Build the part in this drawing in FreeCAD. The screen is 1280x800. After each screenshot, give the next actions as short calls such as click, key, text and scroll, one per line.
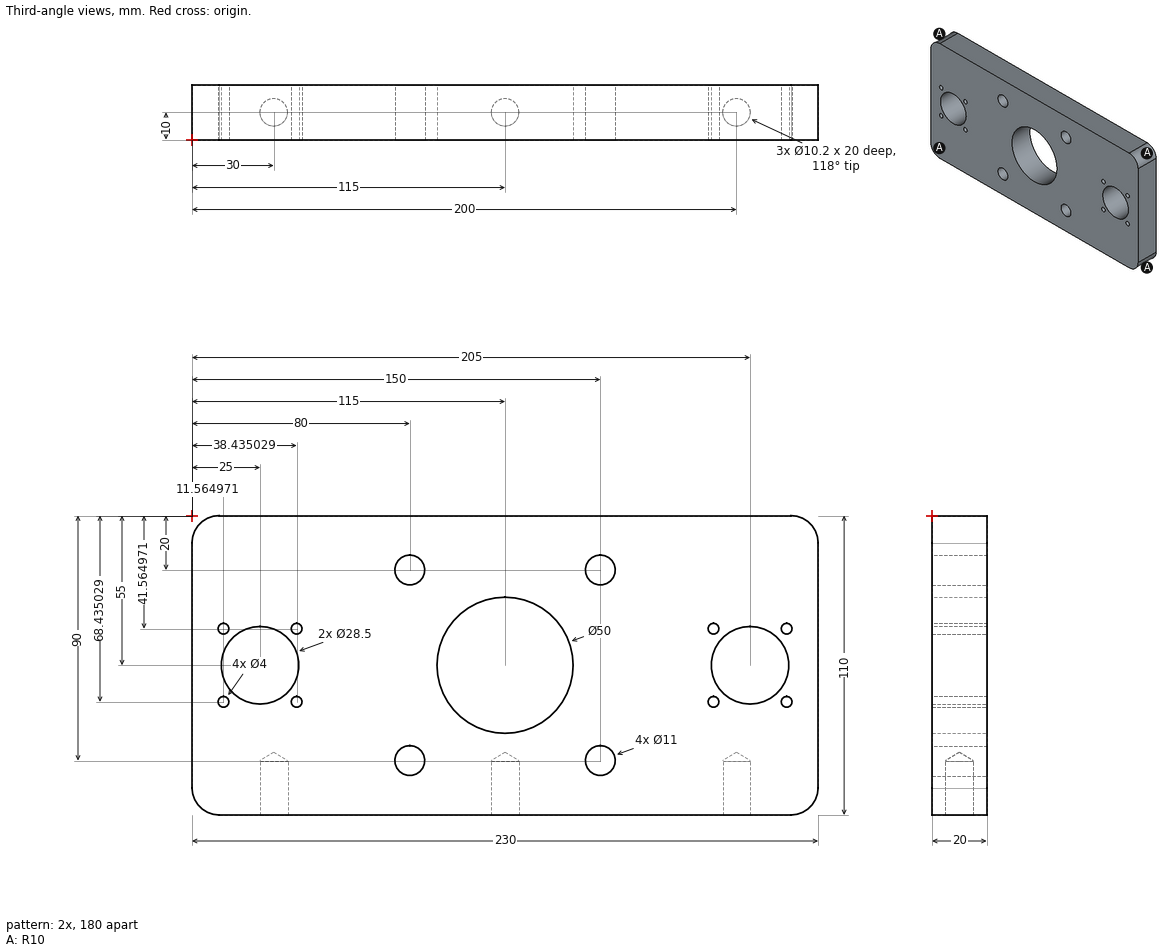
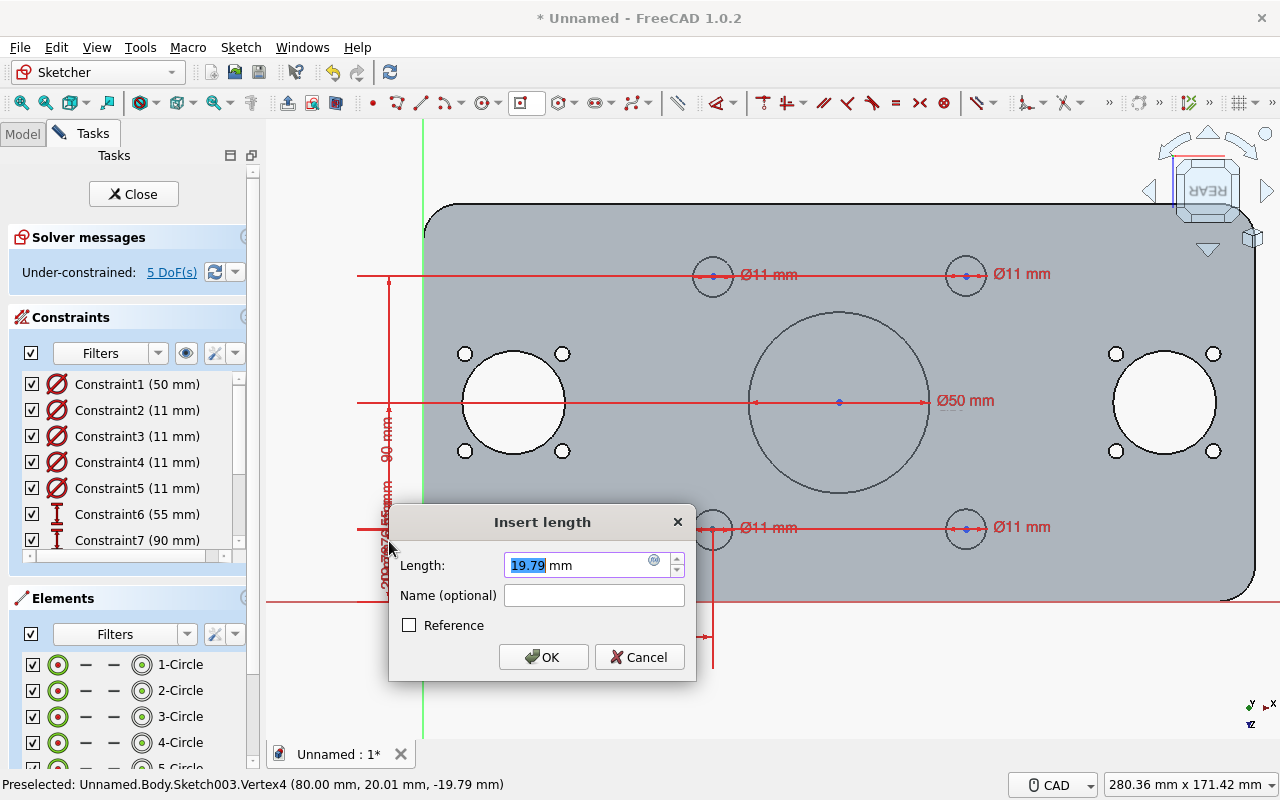
text(20)
key(Return)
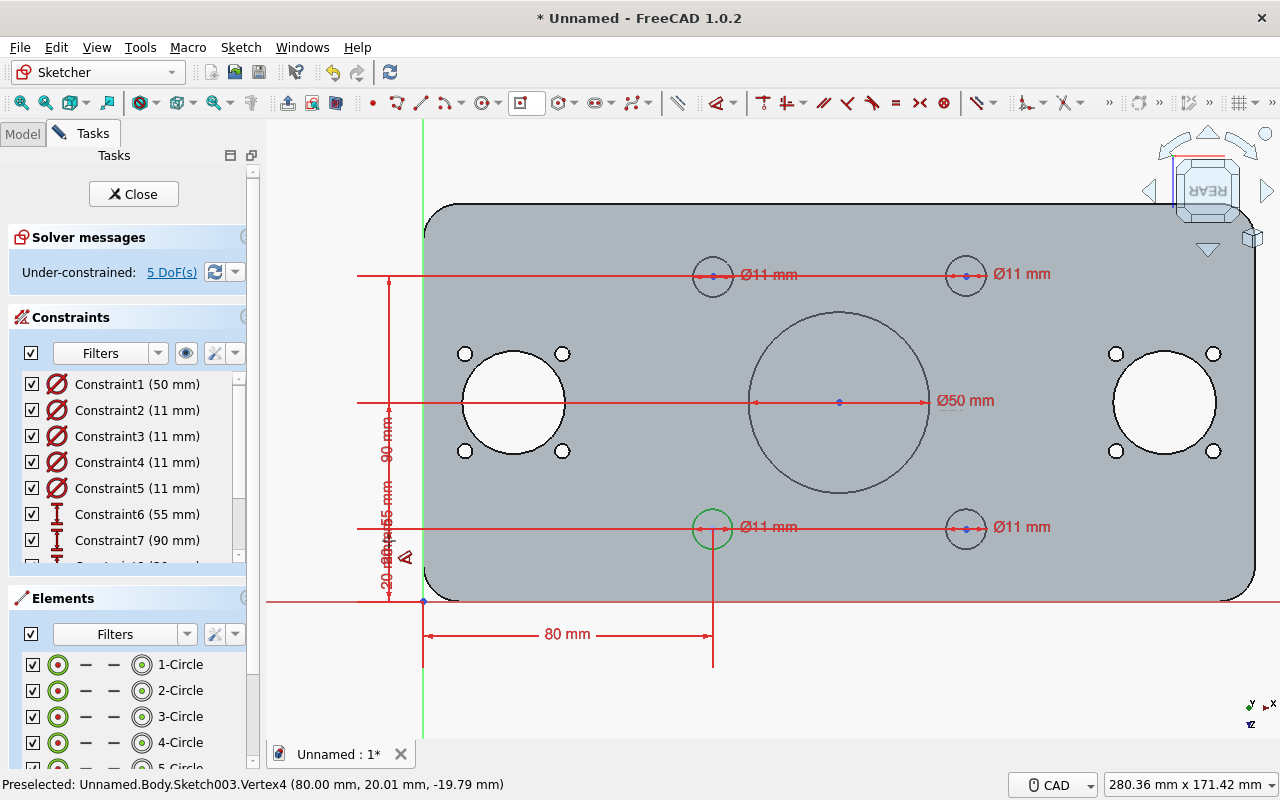
click(713, 277)
click(467, 636)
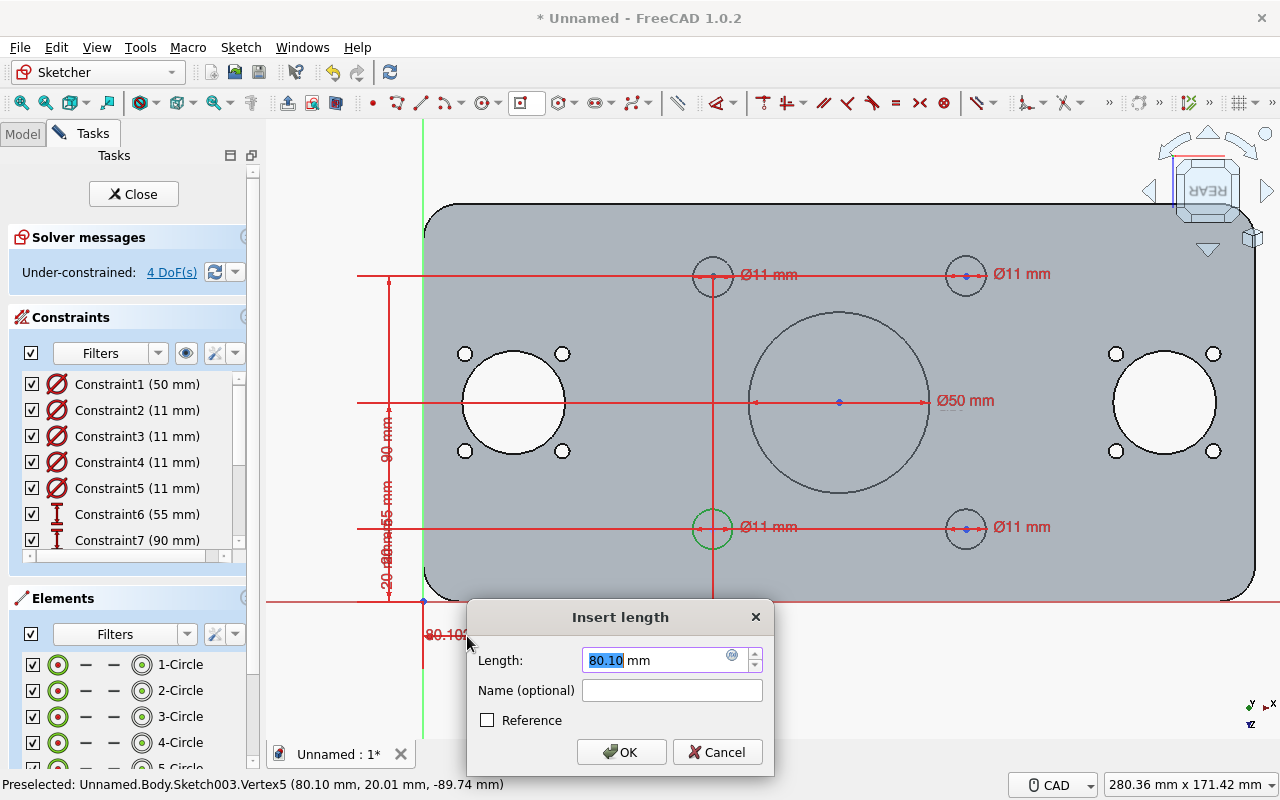
text(80)
key(Return)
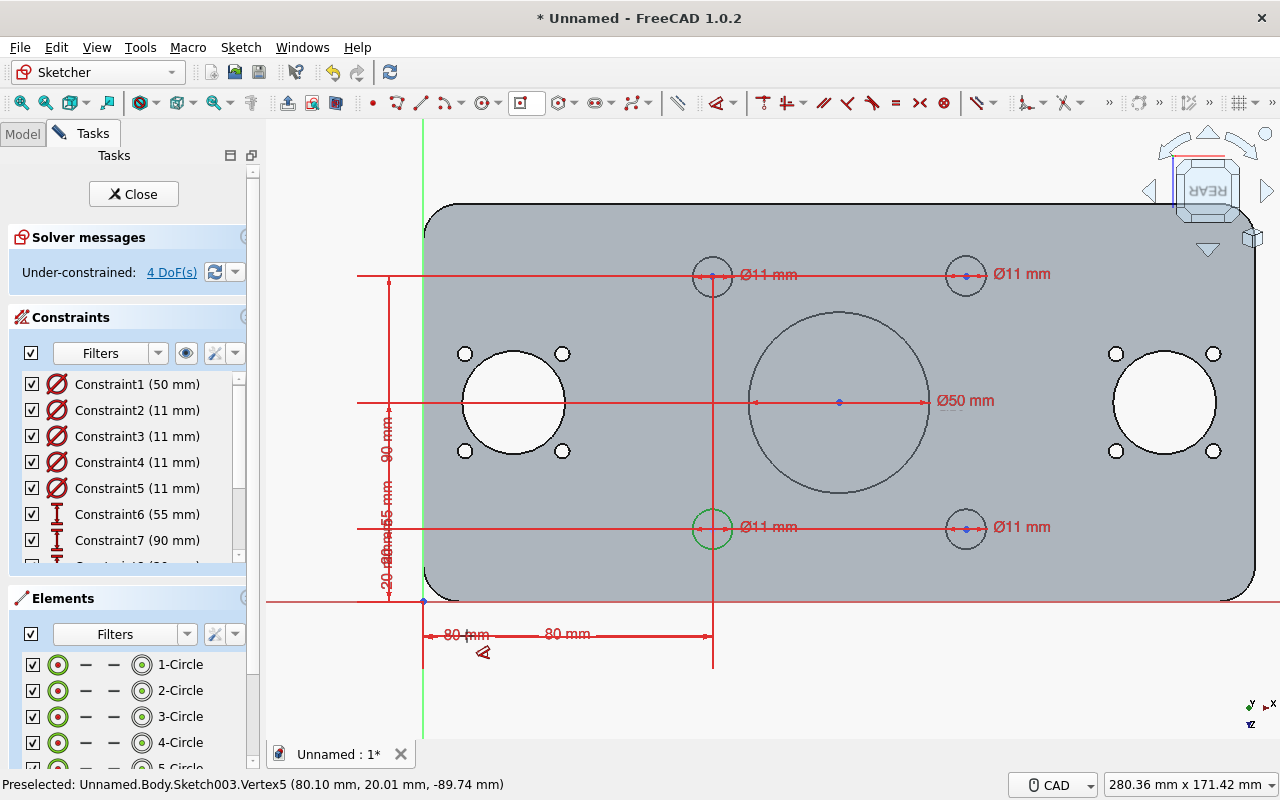
click(713, 277)
click(389, 365)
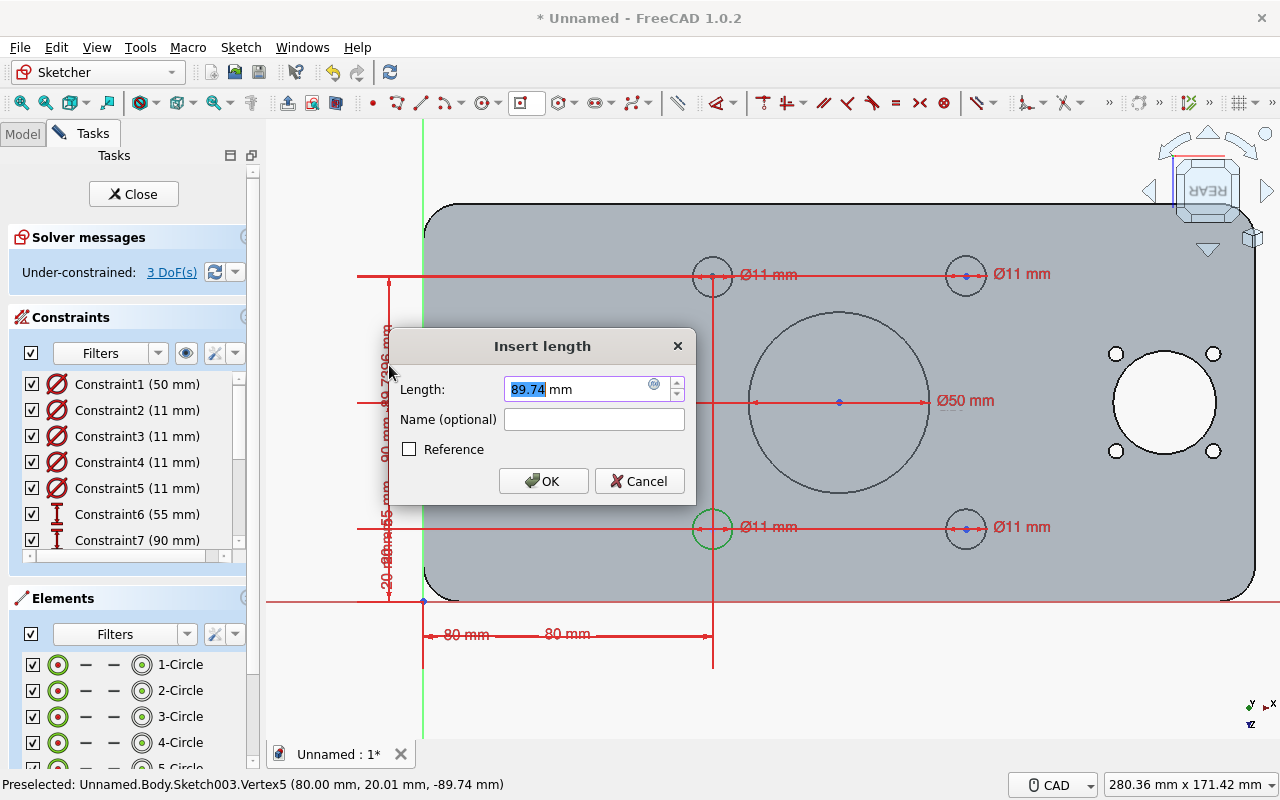
text(90)
key(Return)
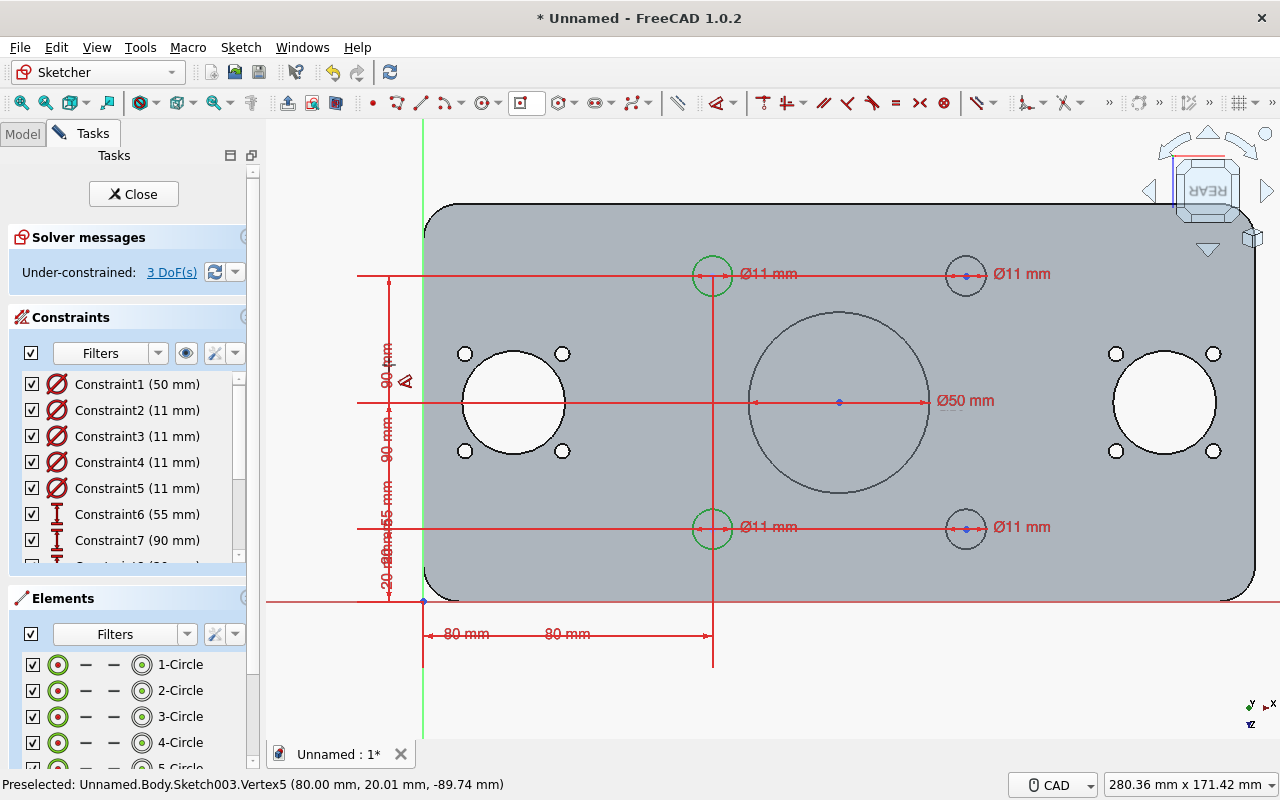
click(839, 403)
click(727, 636)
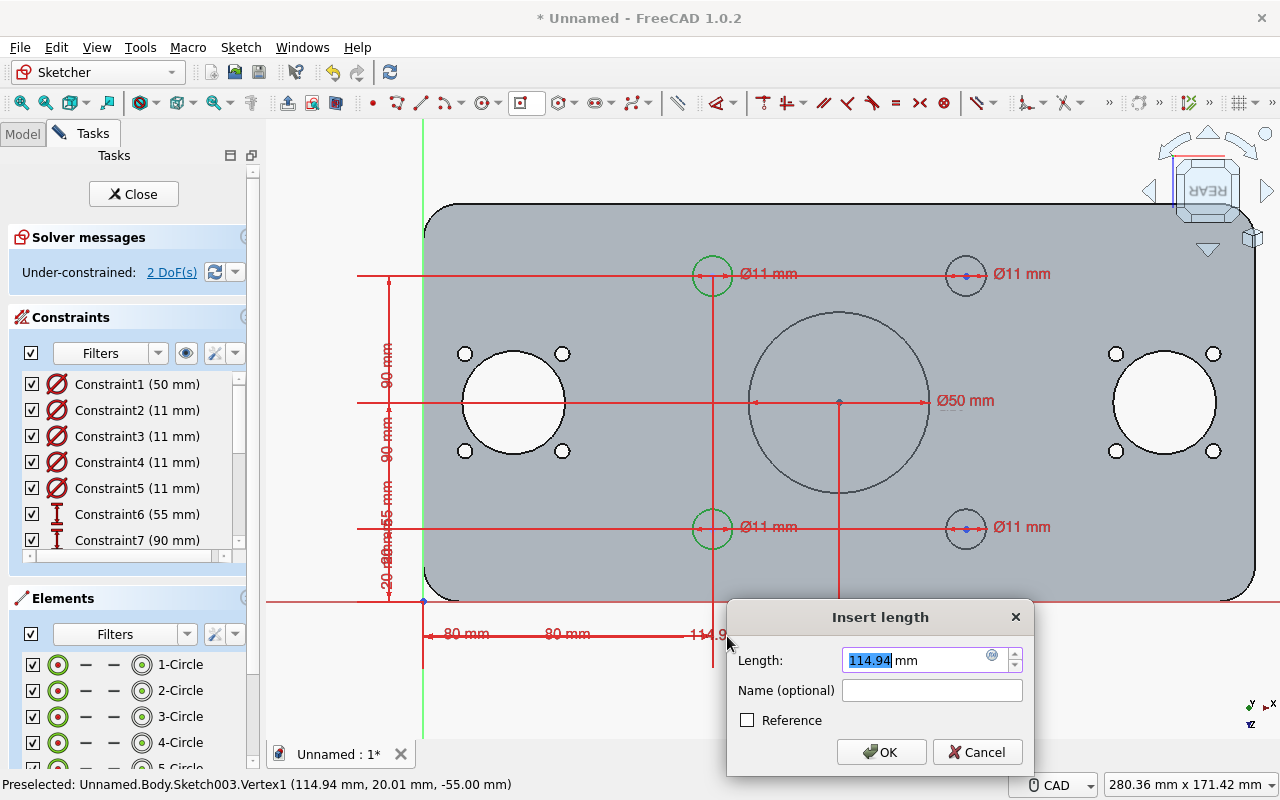
text(115)
key(Return)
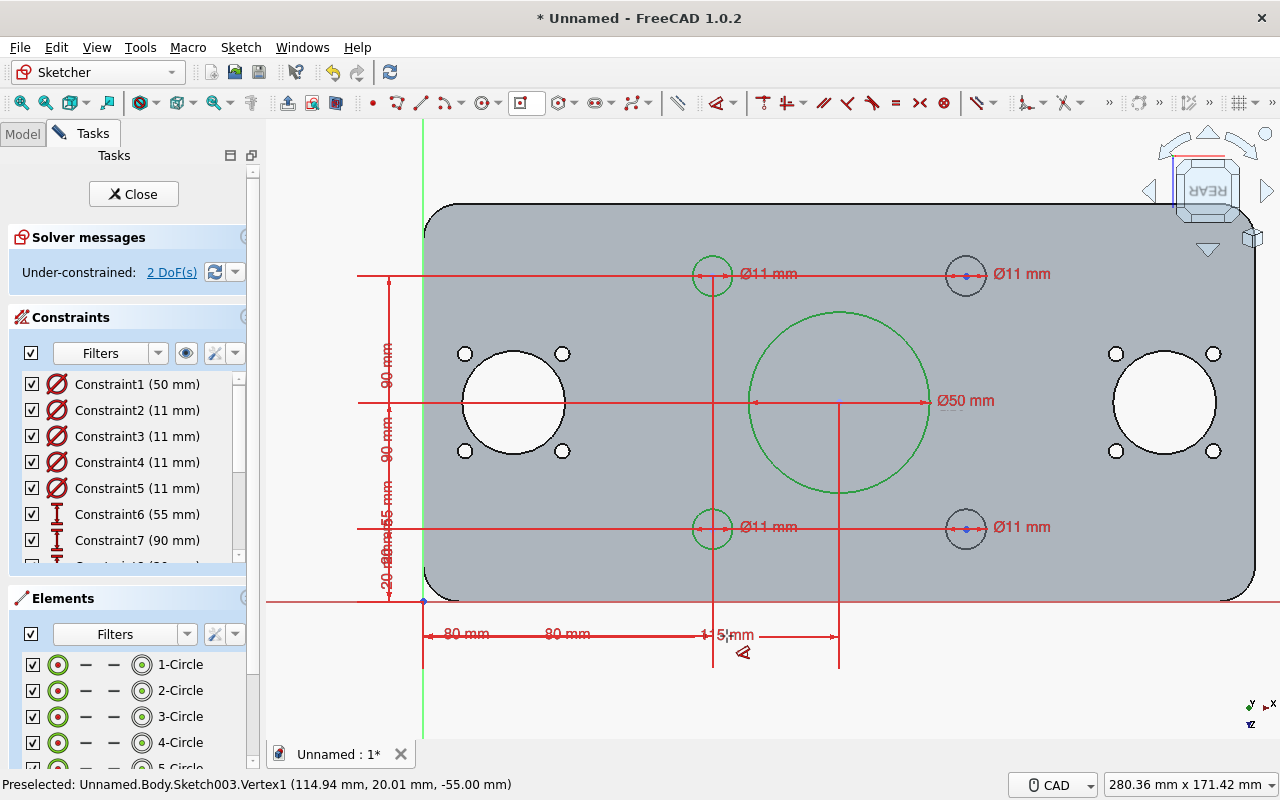
click(966, 276)
click(819, 636)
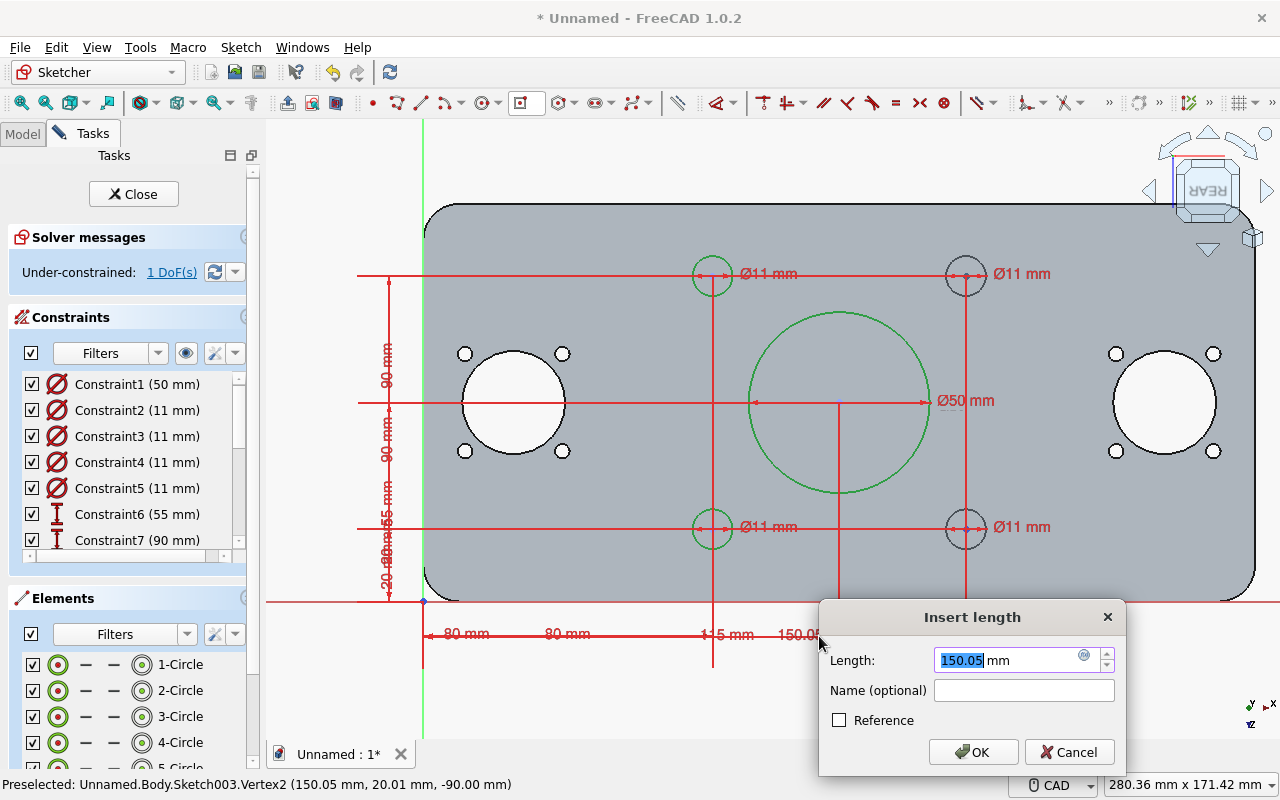
text(150)
key(Return)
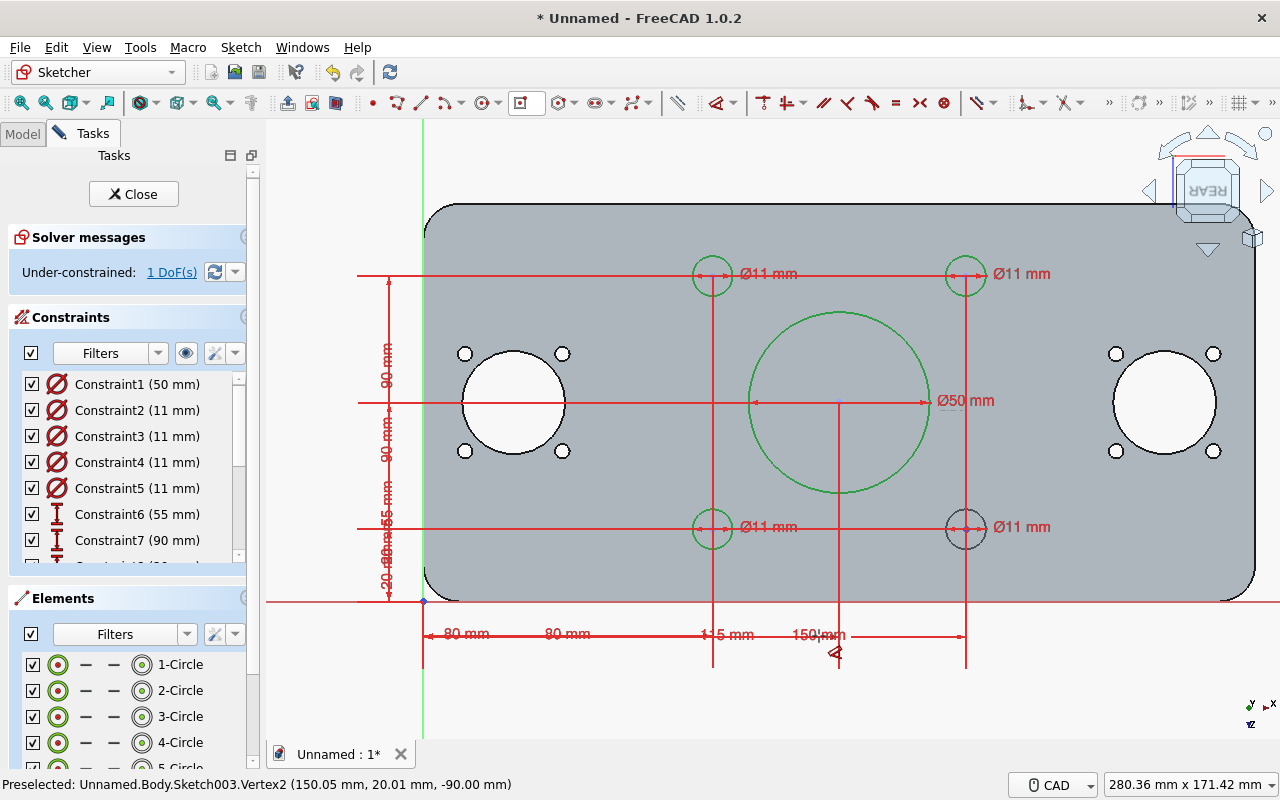
click(966, 529)
click(695, 495)